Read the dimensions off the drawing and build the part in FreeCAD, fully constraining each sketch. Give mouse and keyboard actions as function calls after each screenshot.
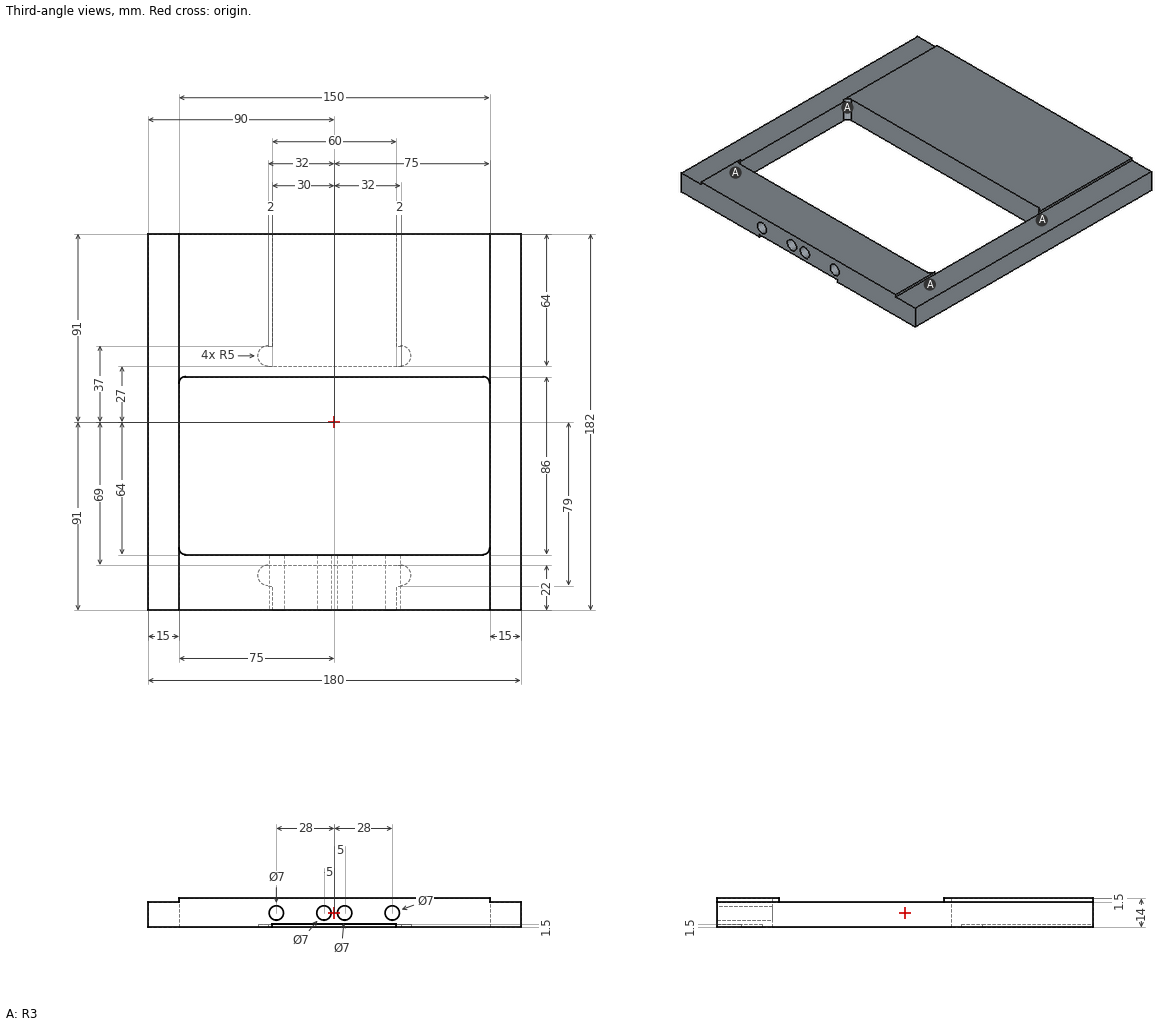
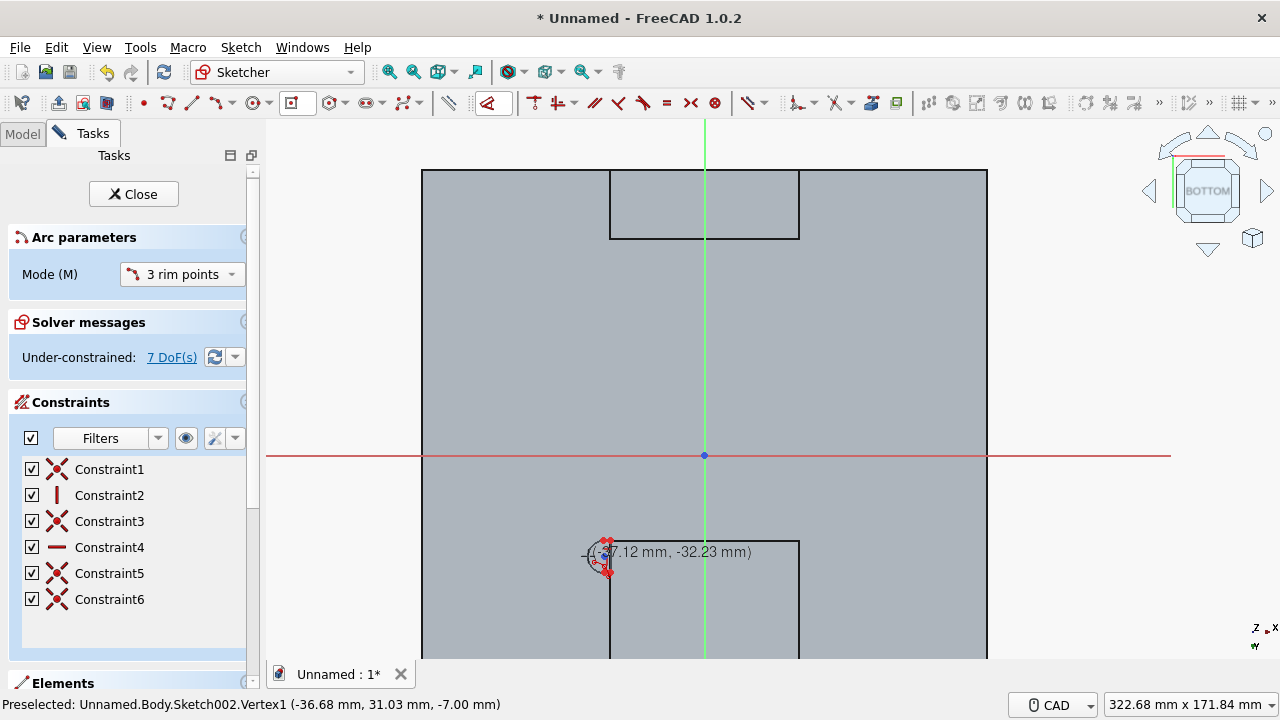
key(g)
key(m)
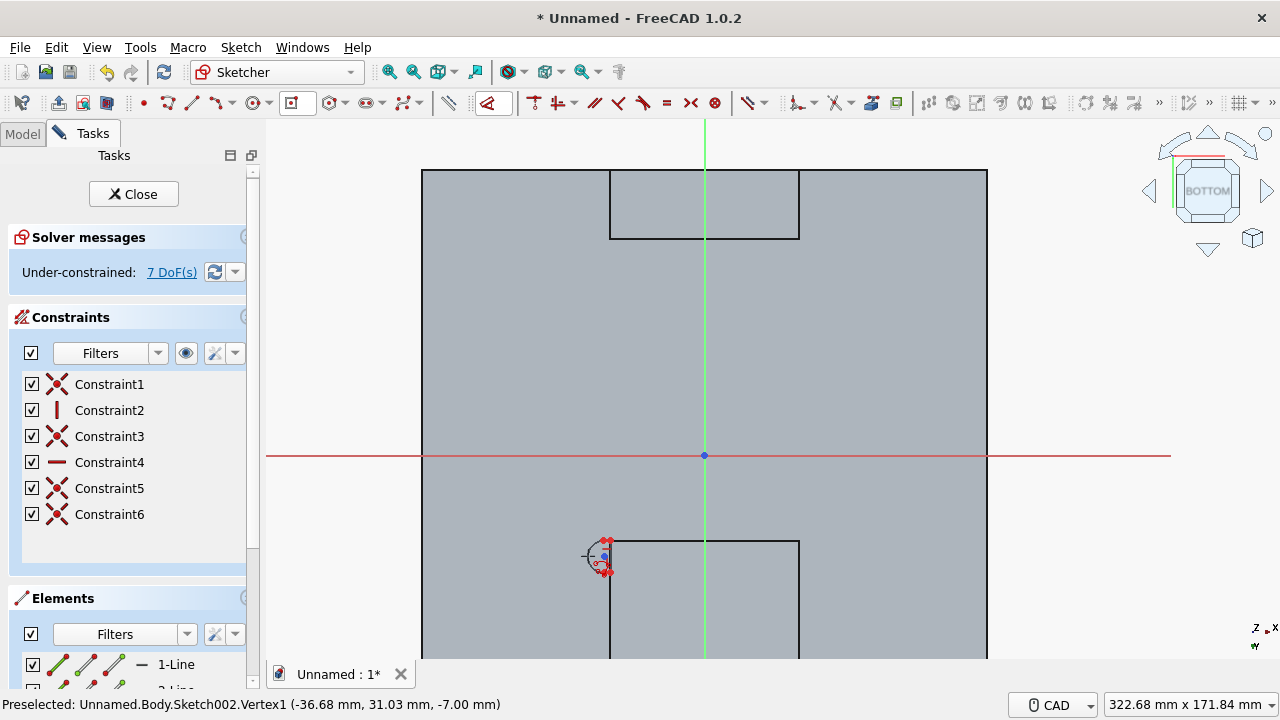
click(805, 541)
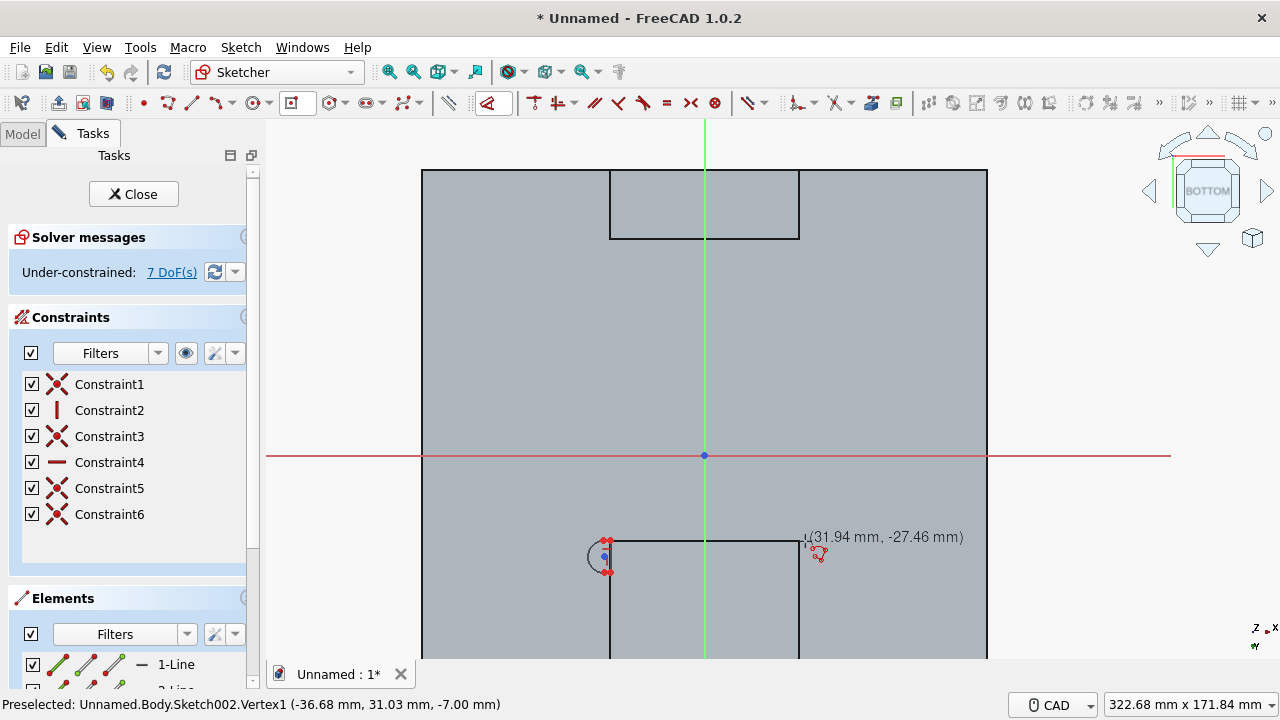
scroll(799, 541, up, 5)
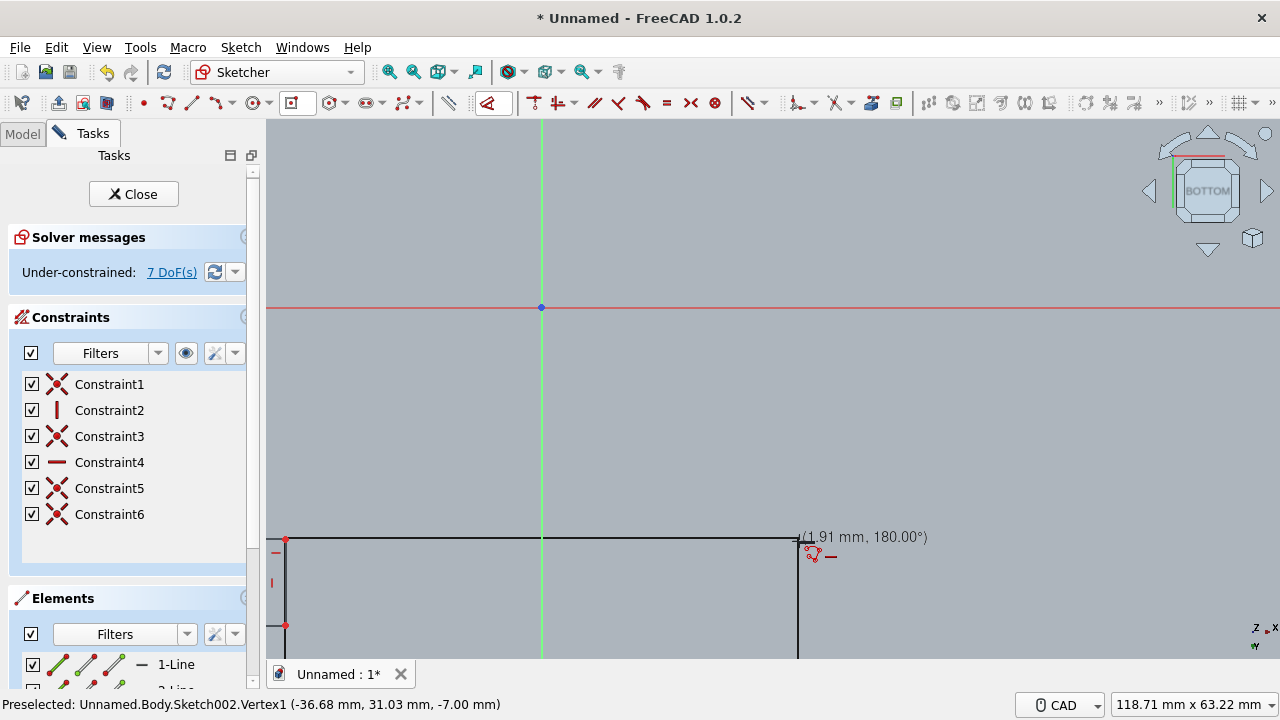
click(798, 540)
click(798, 624)
click(815, 624)
right_click(815, 624)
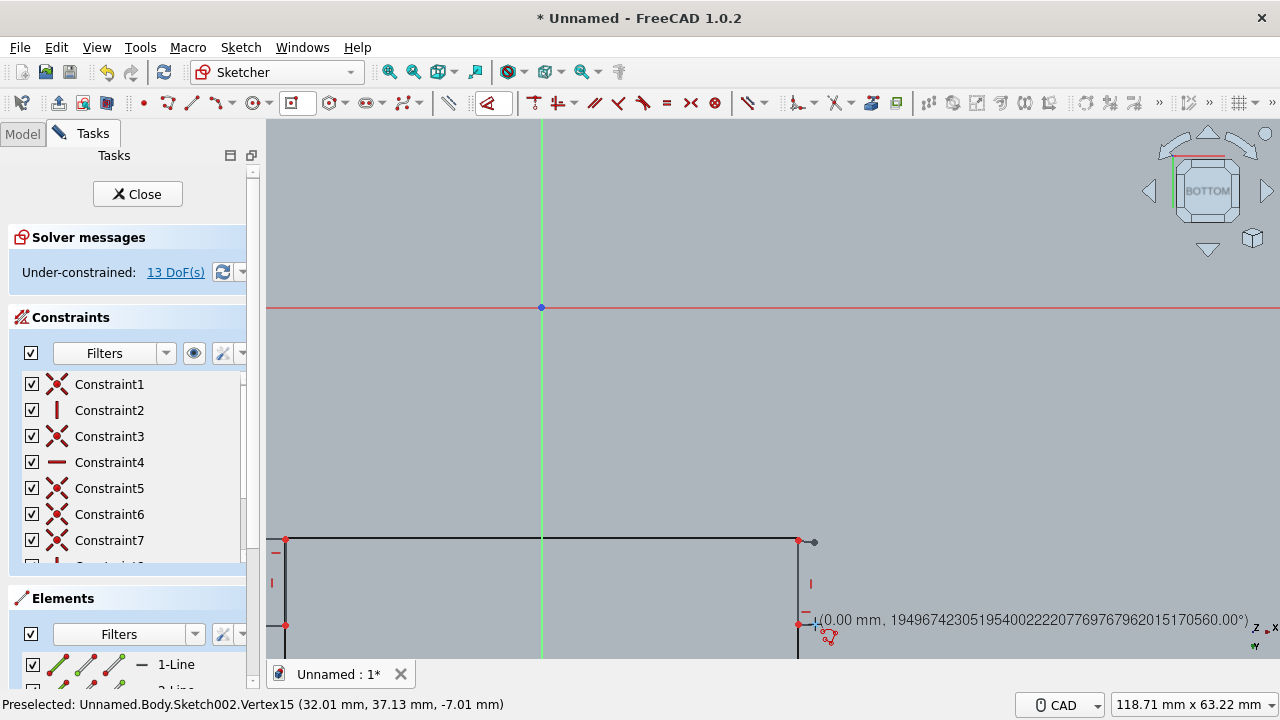
key(g)
key(3)
key(a)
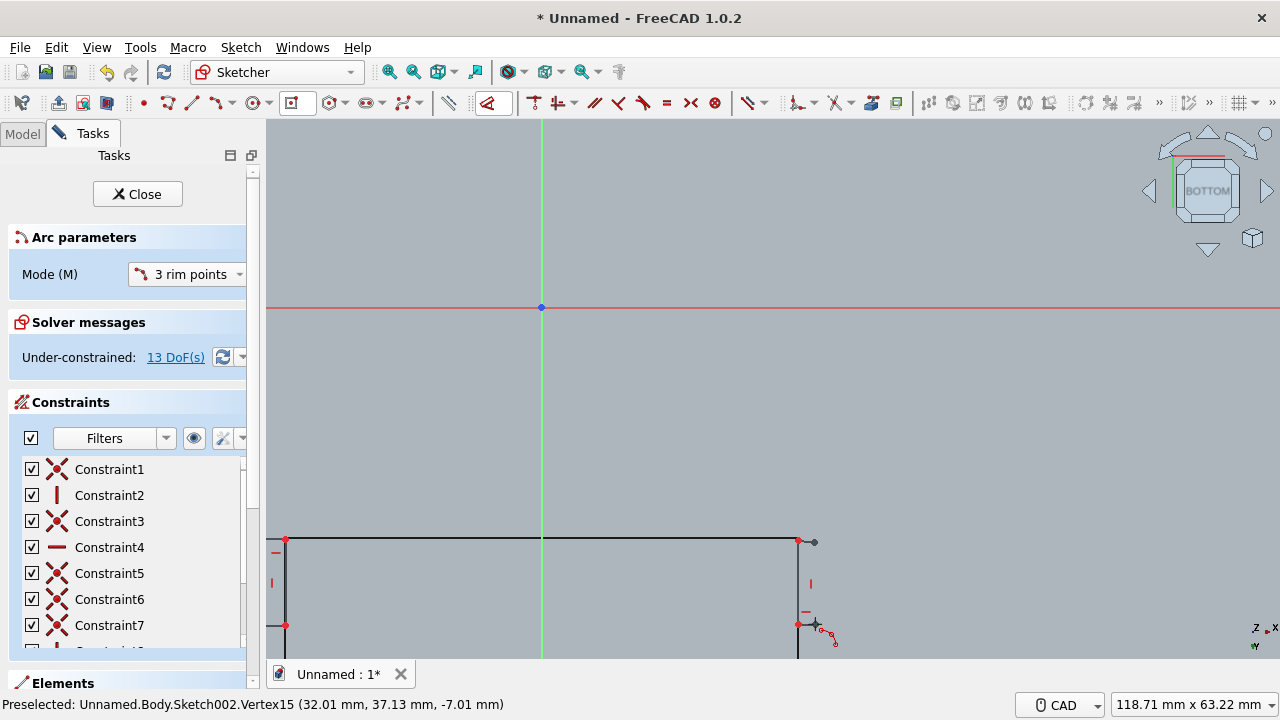
scroll(815, 624, up, 4)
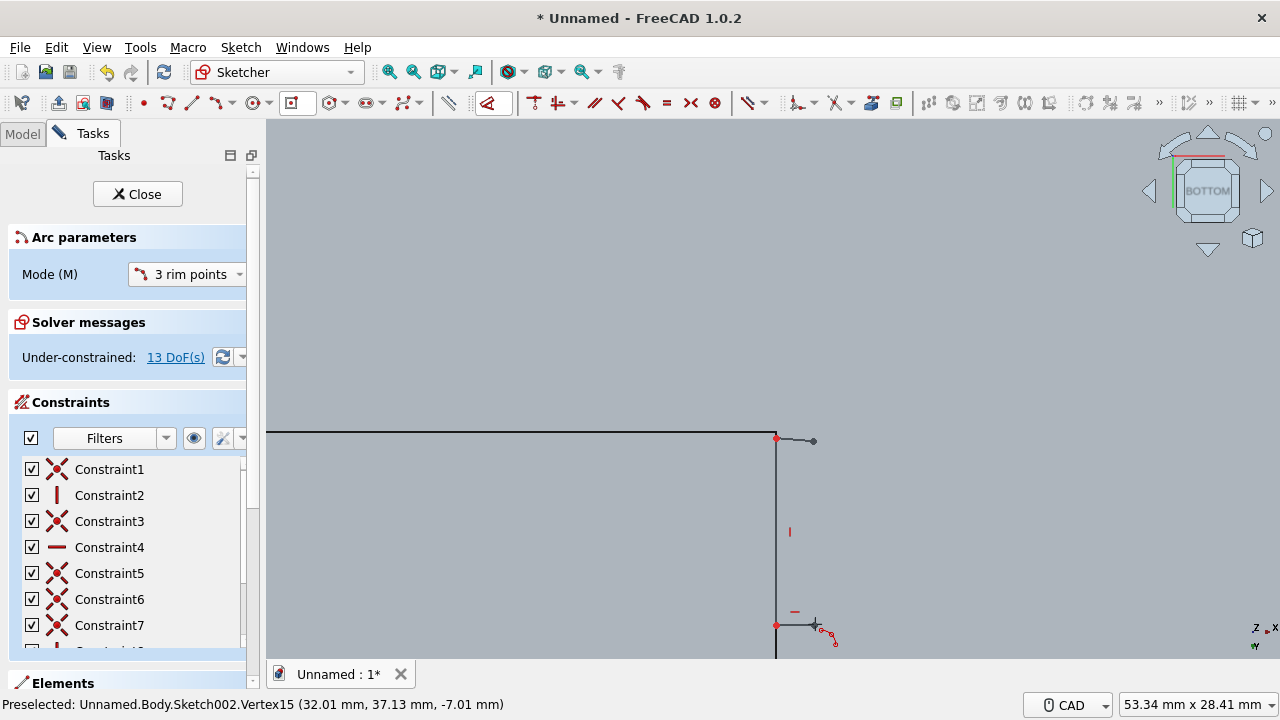
click(814, 625)
click(813, 441)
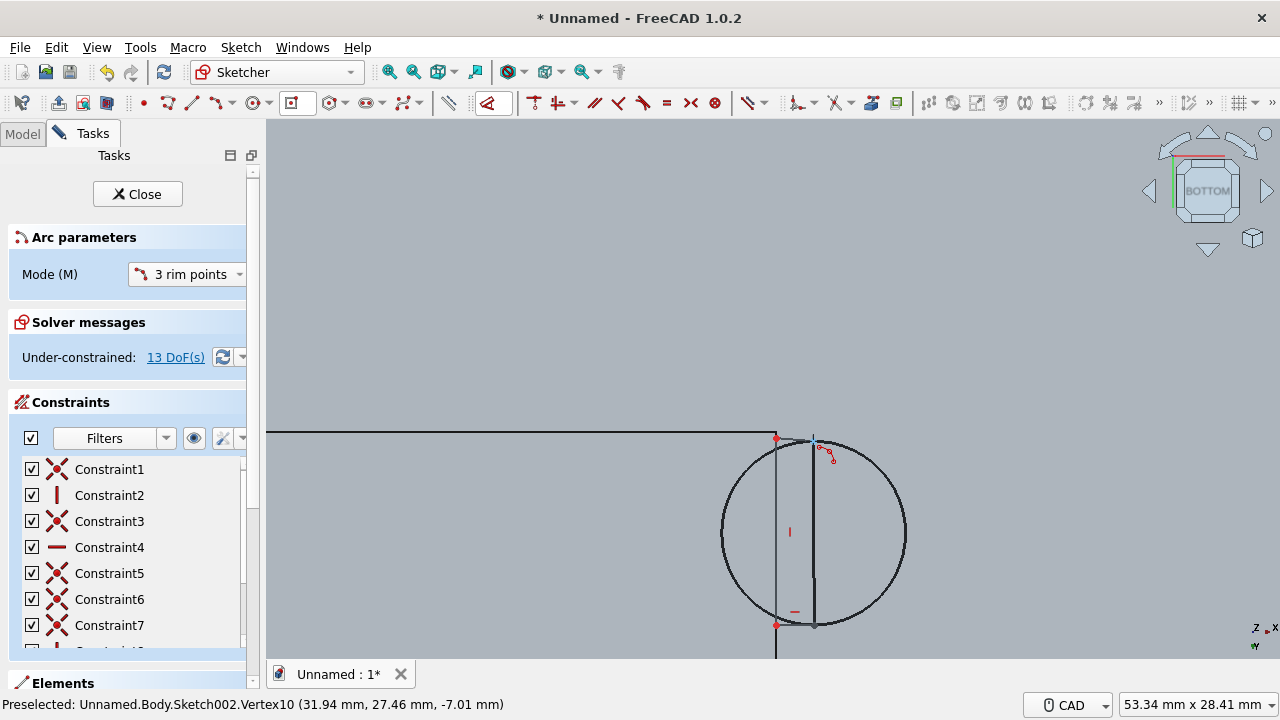
scroll(803, 561, down, 9)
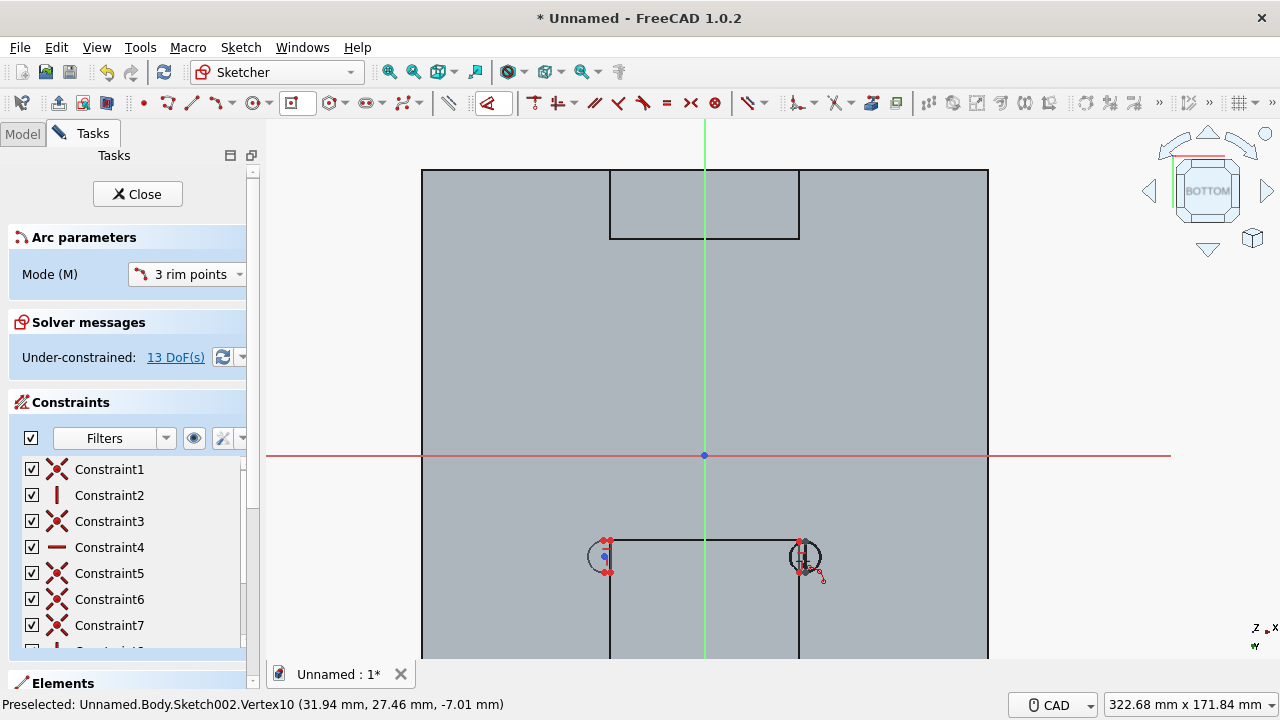
click(821, 556)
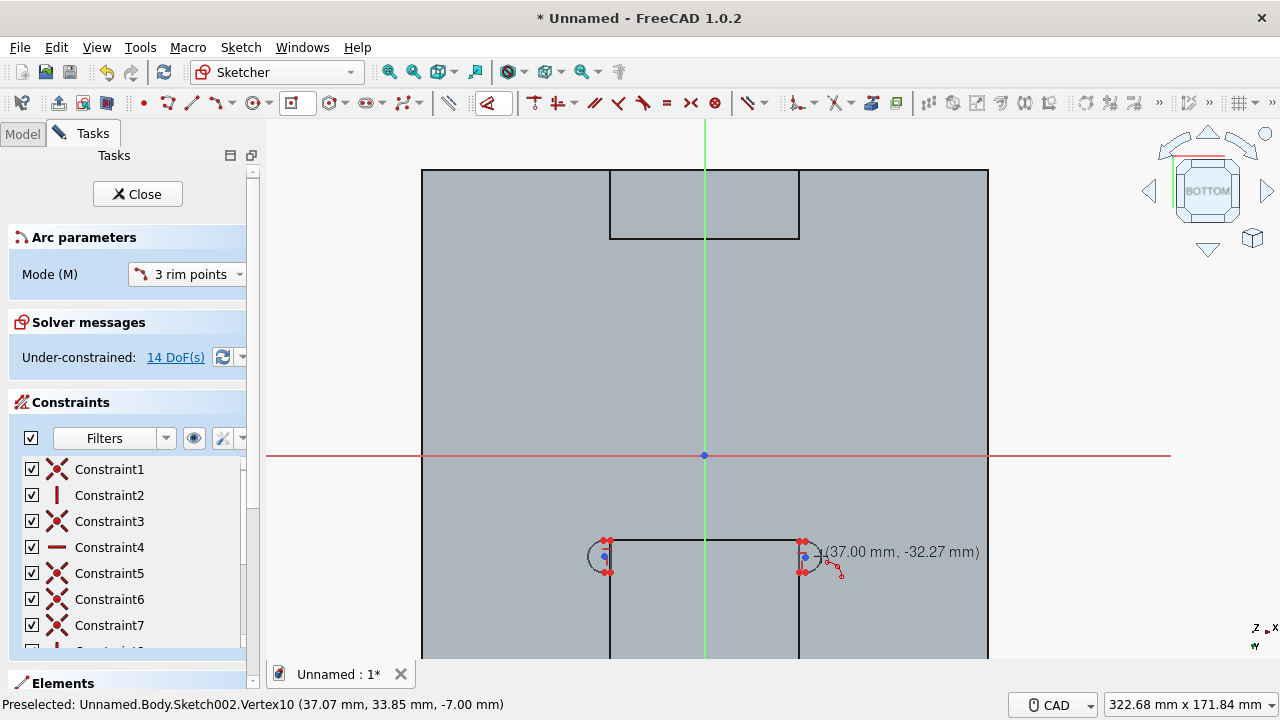
click(168, 104)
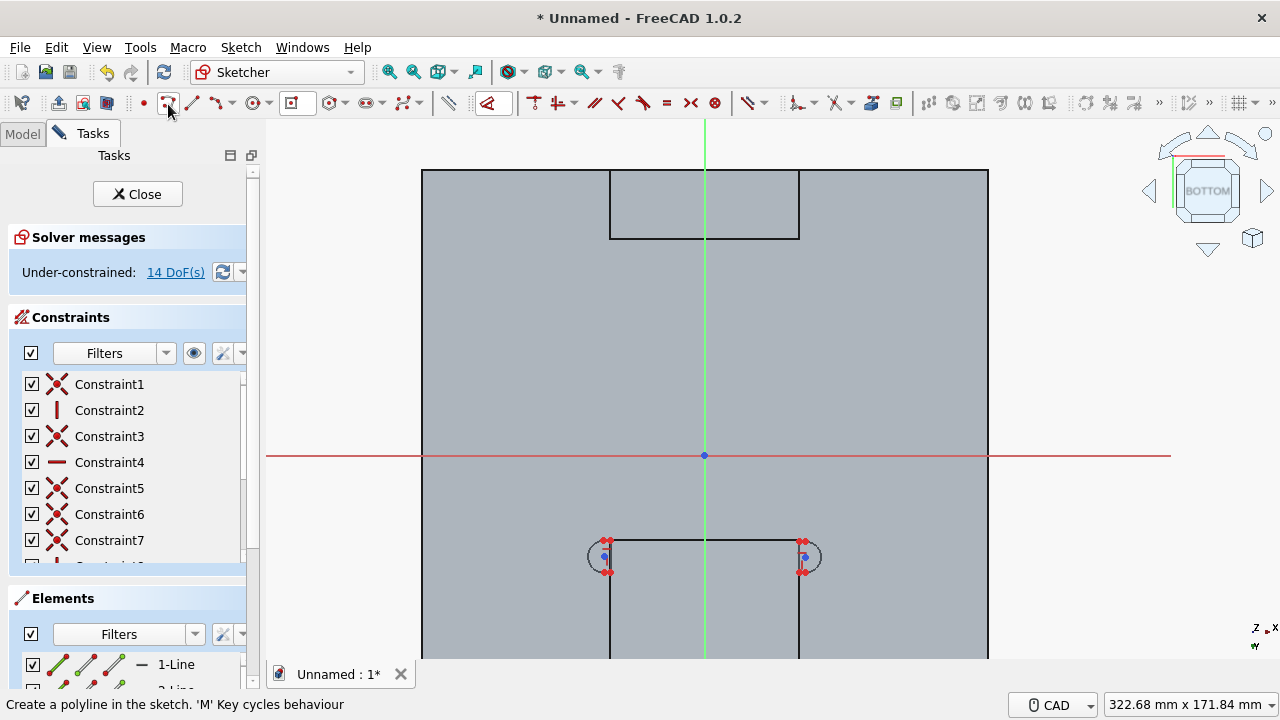
click(604, 239)